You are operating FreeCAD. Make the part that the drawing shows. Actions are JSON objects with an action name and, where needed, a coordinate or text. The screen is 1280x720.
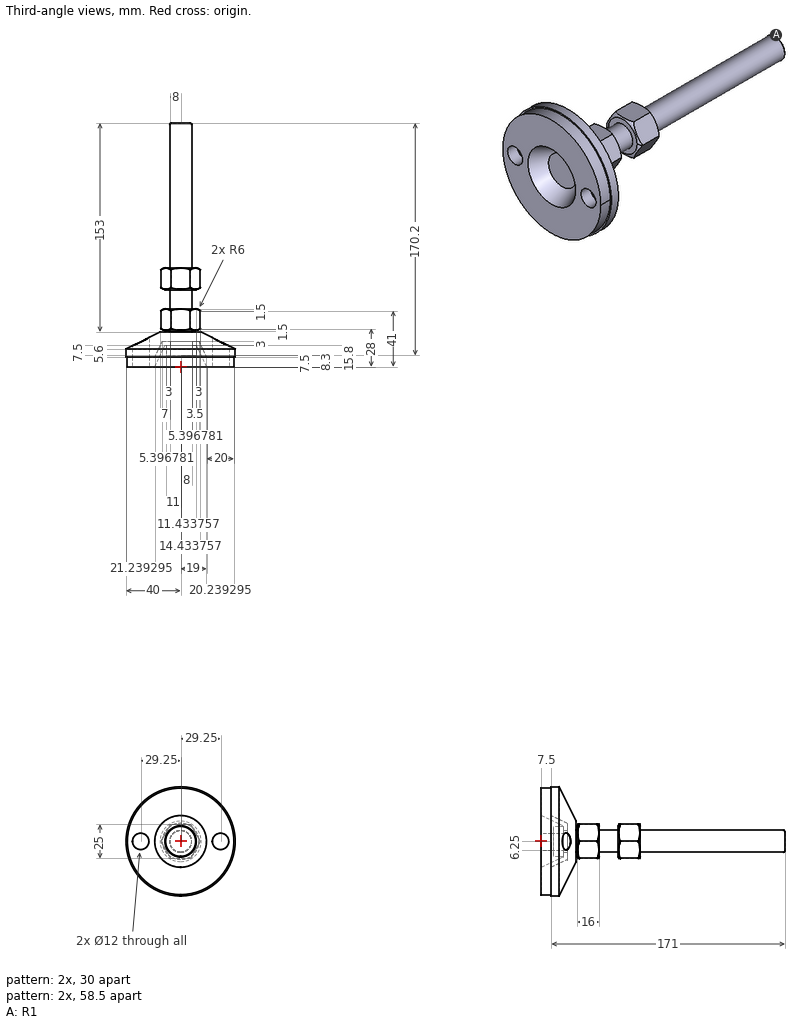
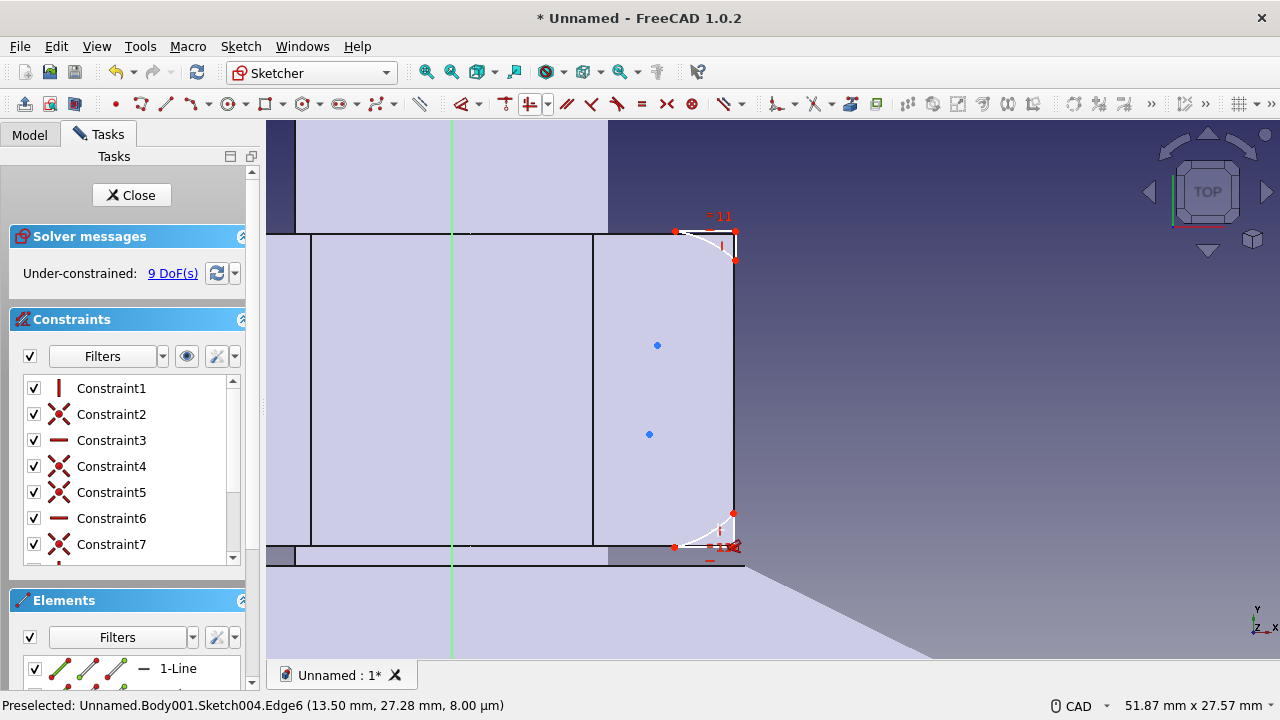
{"action": "left_click", "coordinate": [720, 248]}
{"action": "left_click", "coordinate": [787, 275]}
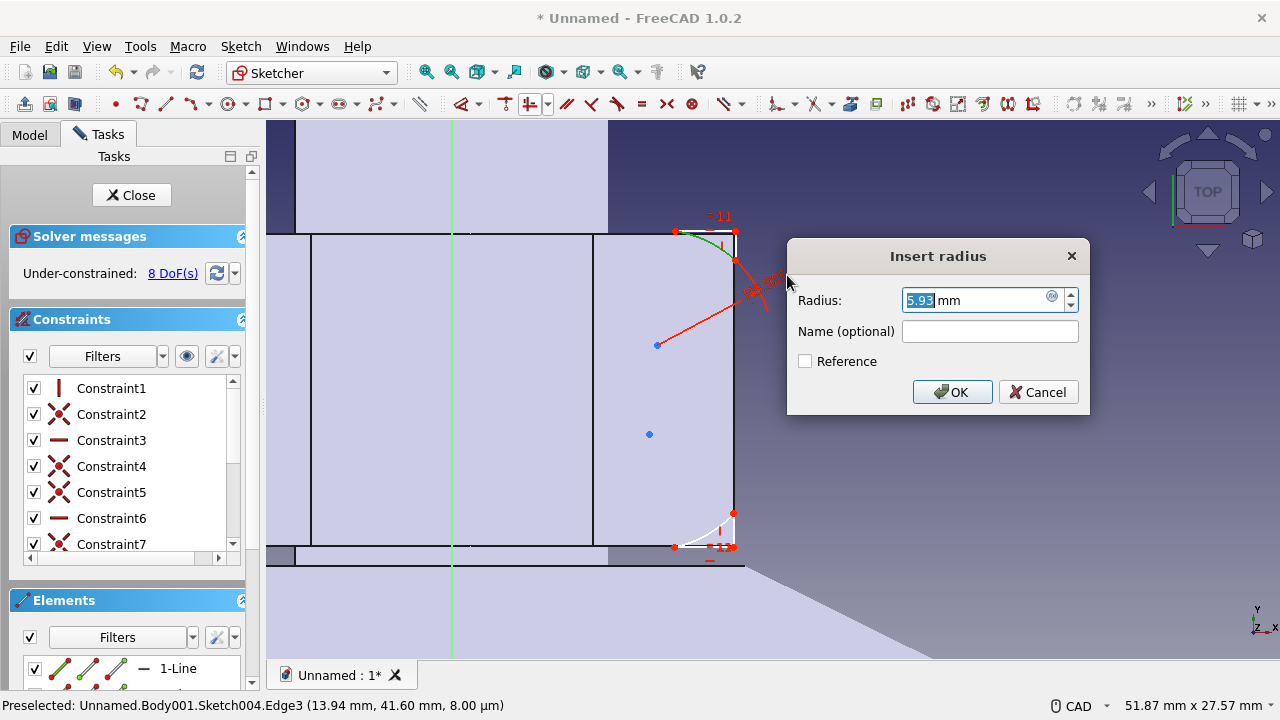
{"action": "type", "text": "6"}
{"action": "key", "text": "Return"}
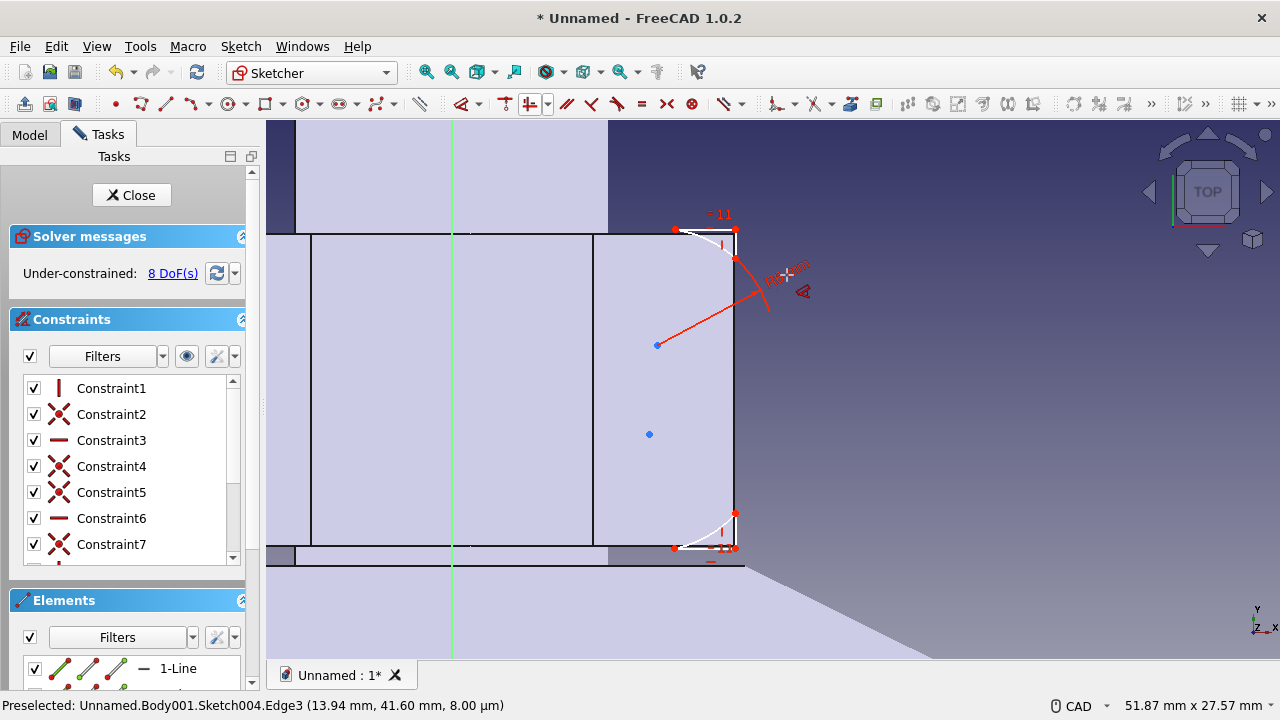
{"action": "left_click", "coordinate": [718, 230]}
{"action": "left_click", "coordinate": [706, 196]}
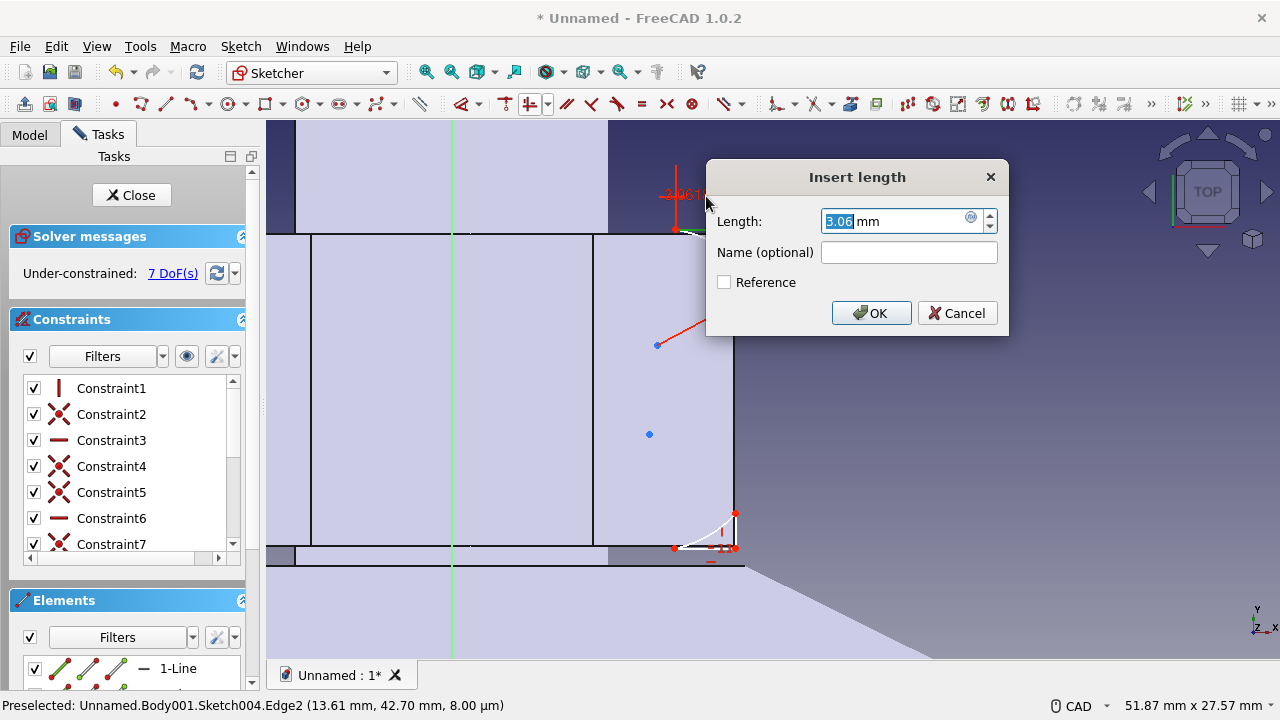
{"action": "type", "text": "3"}
{"action": "key", "text": "Return"}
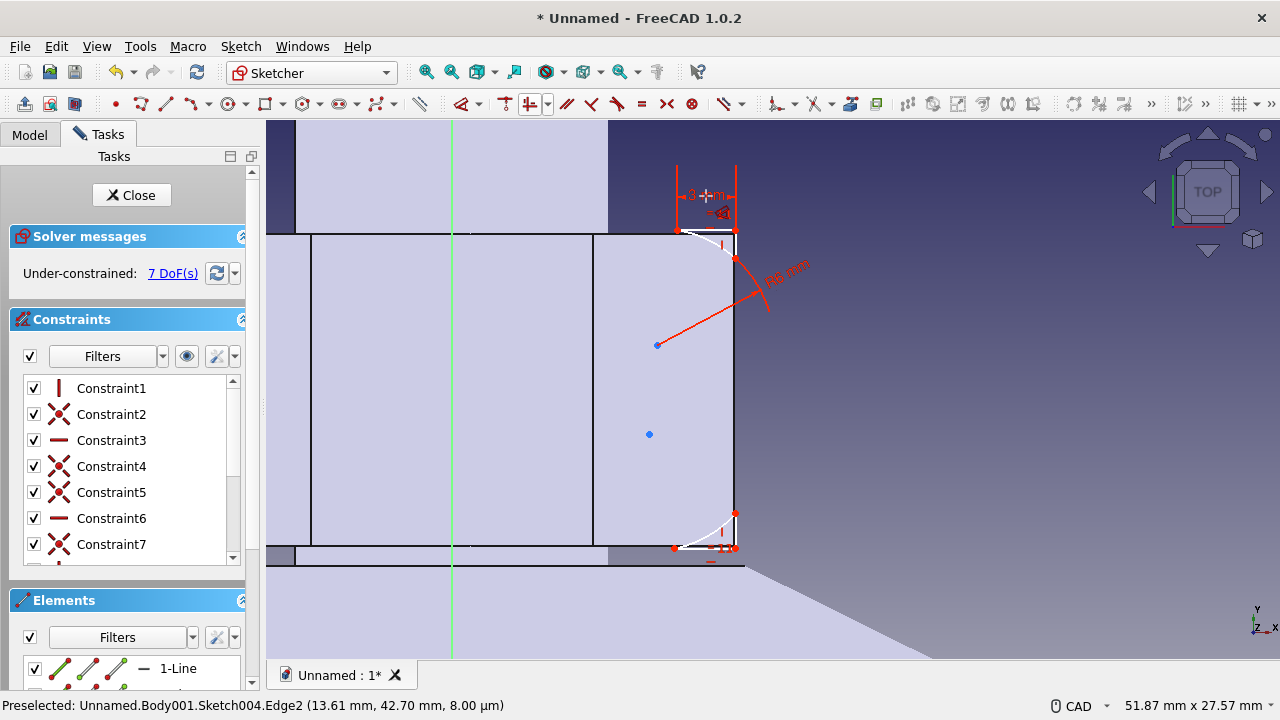
{"action": "left_click", "coordinate": [718, 549]}
{"action": "left_click", "coordinate": [705, 583]}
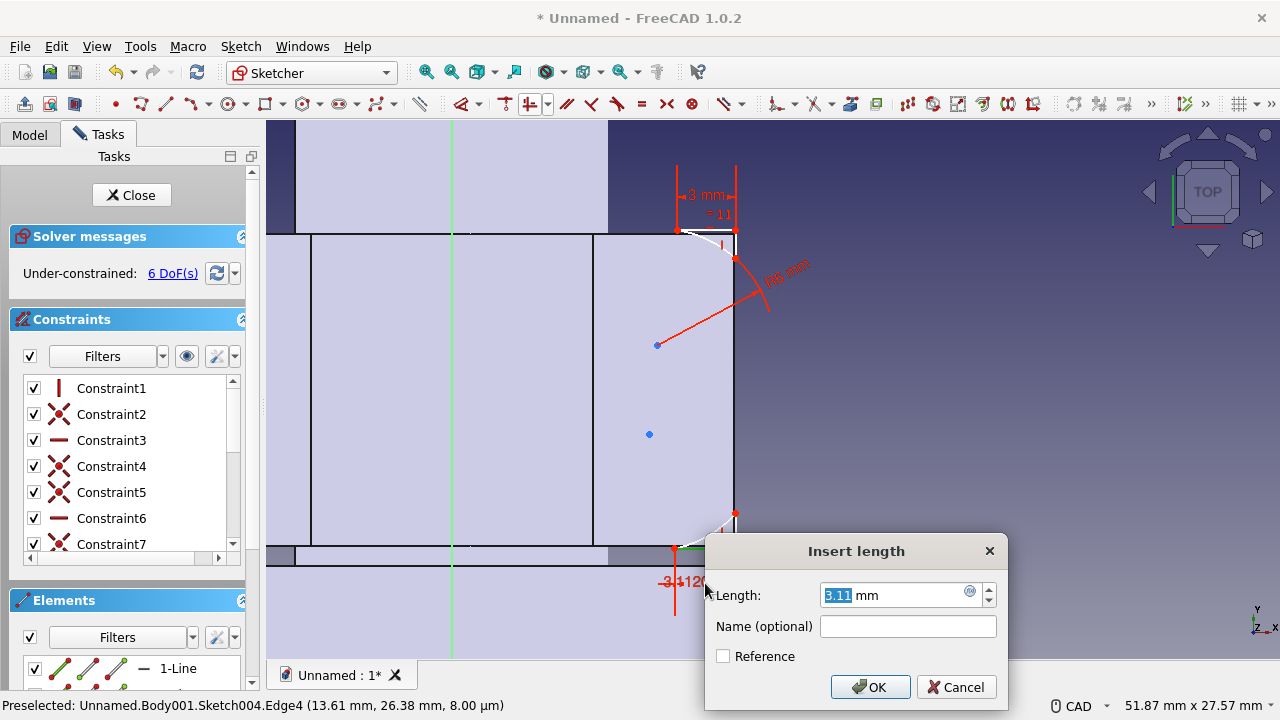
{"action": "type", "text": "3"}
{"action": "key", "text": "Return"}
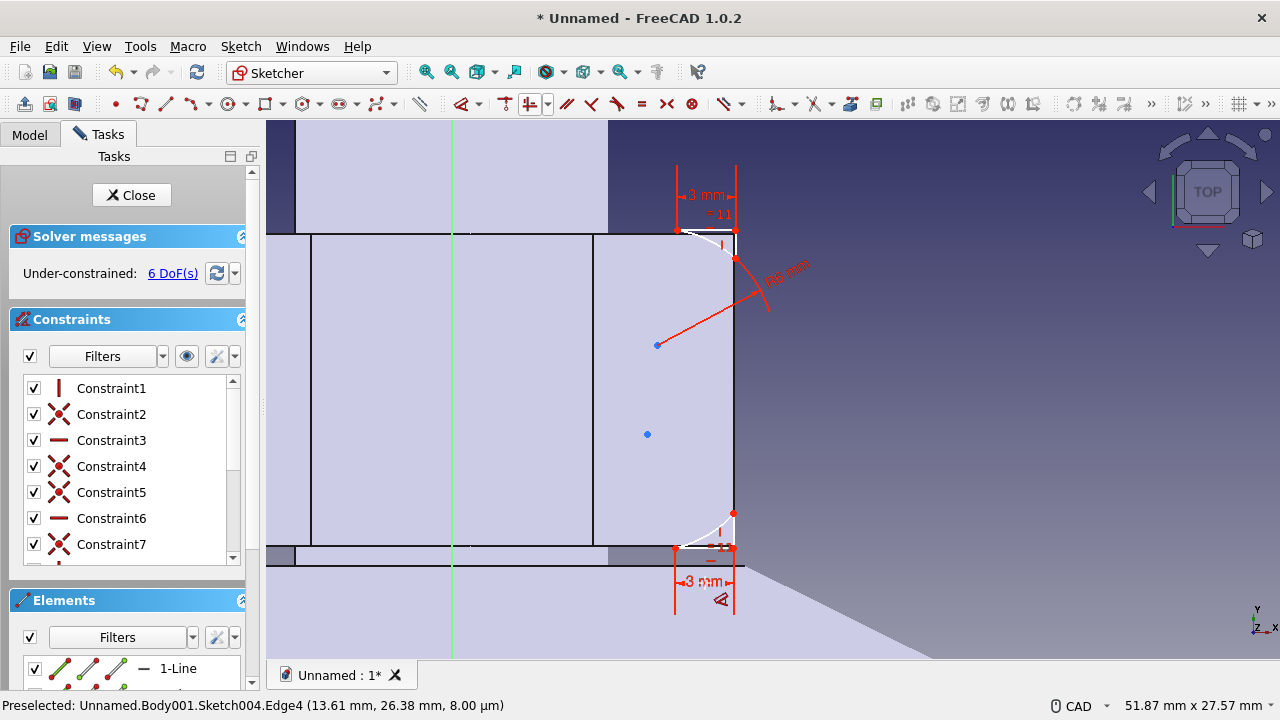
{"action": "scroll", "coordinate": [736, 241], "scroll_direction": "up", "scroll_amount": 2}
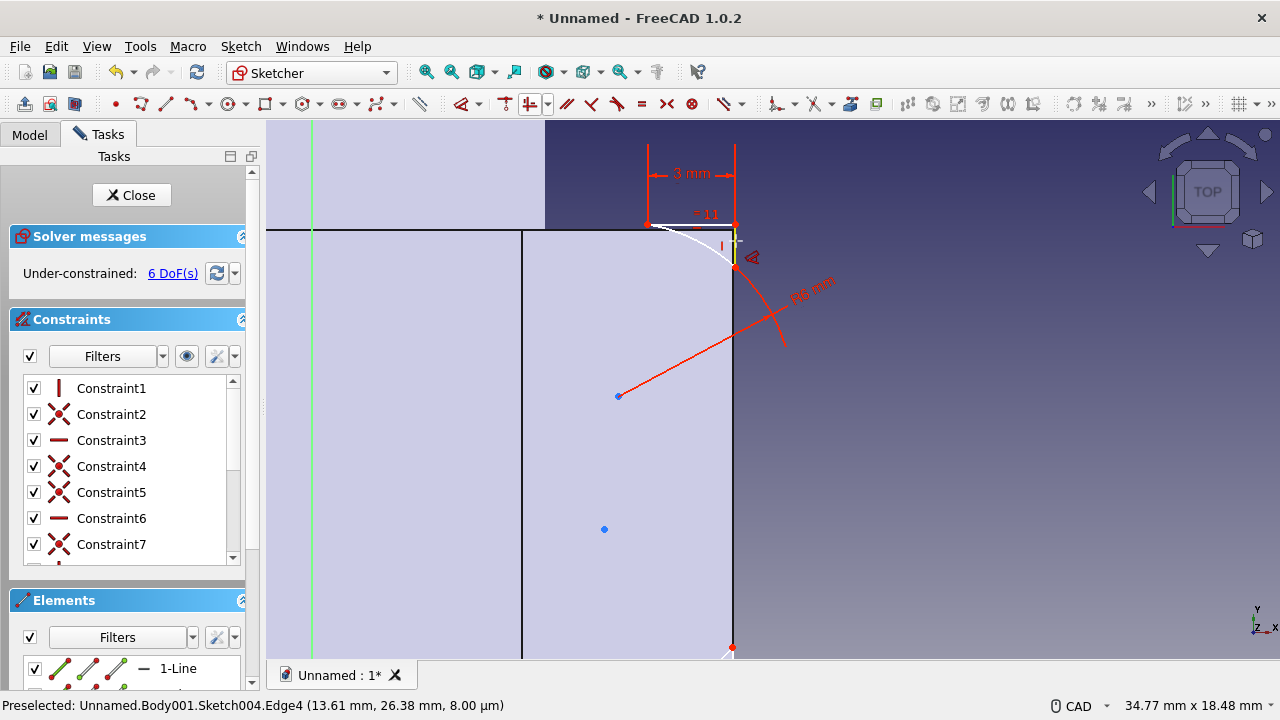
{"action": "left_click", "coordinate": [735, 242]}
{"action": "left_click", "coordinate": [769, 246]}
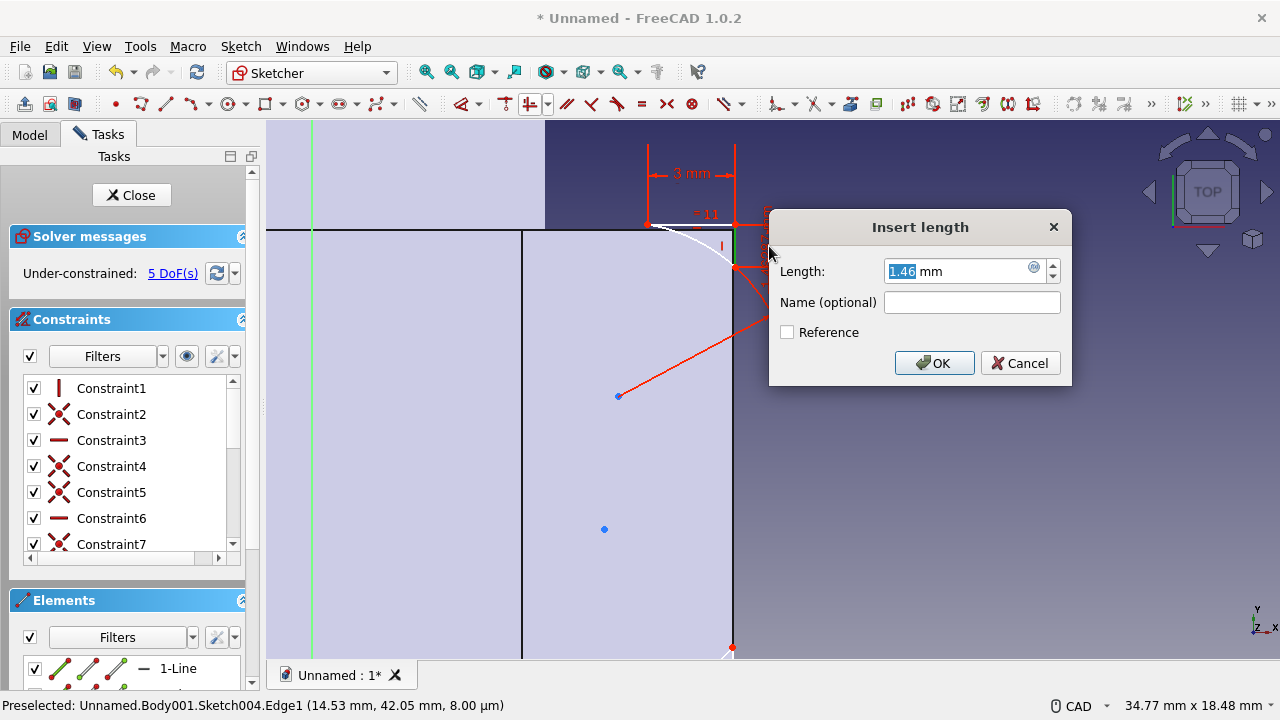
{"action": "type", "text": "1.5"}
{"action": "key", "text": "Return"}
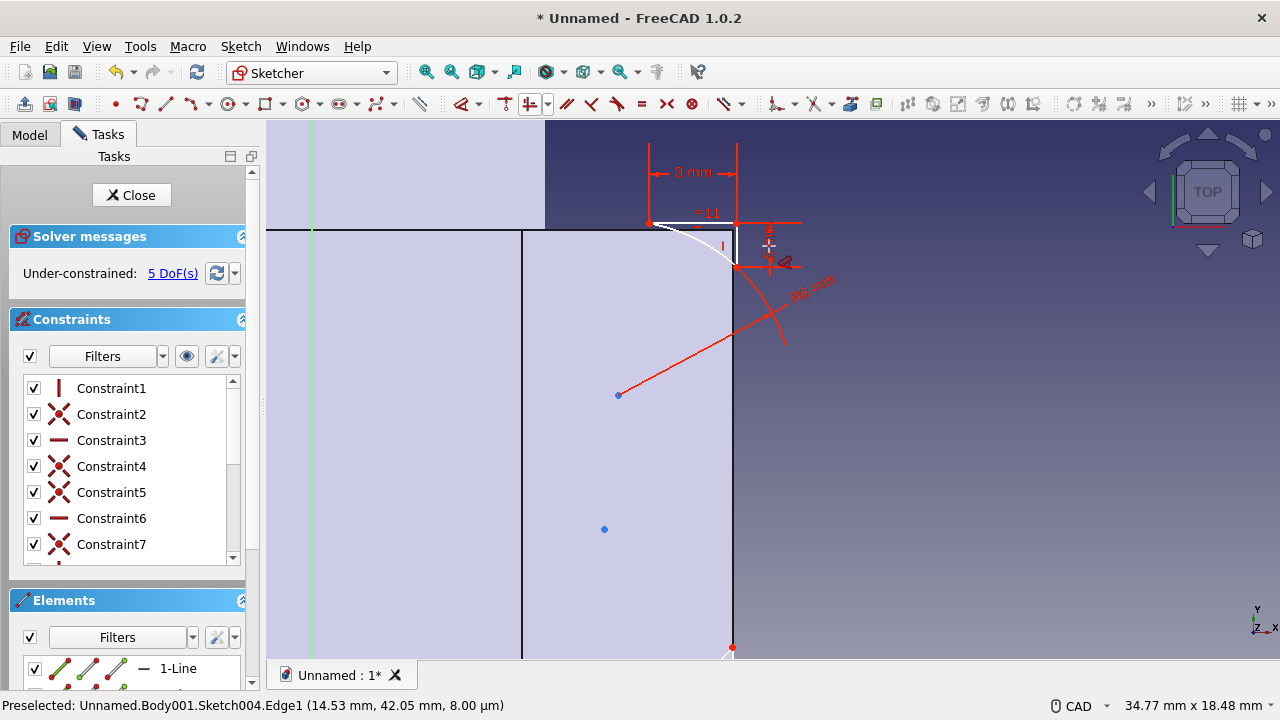
{"action": "scroll", "coordinate": [736, 240], "scroll_direction": "down", "scroll_amount": 2}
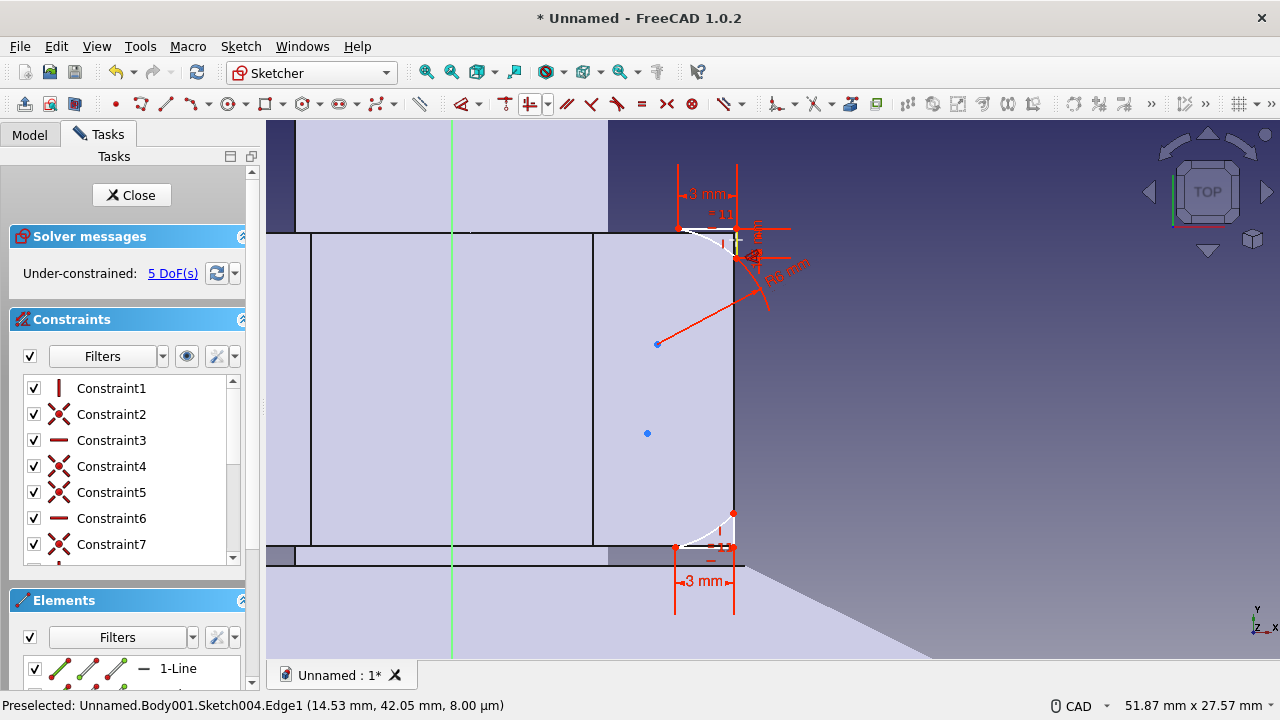
{"action": "scroll", "coordinate": [734, 538], "scroll_direction": "up", "scroll_amount": 2}